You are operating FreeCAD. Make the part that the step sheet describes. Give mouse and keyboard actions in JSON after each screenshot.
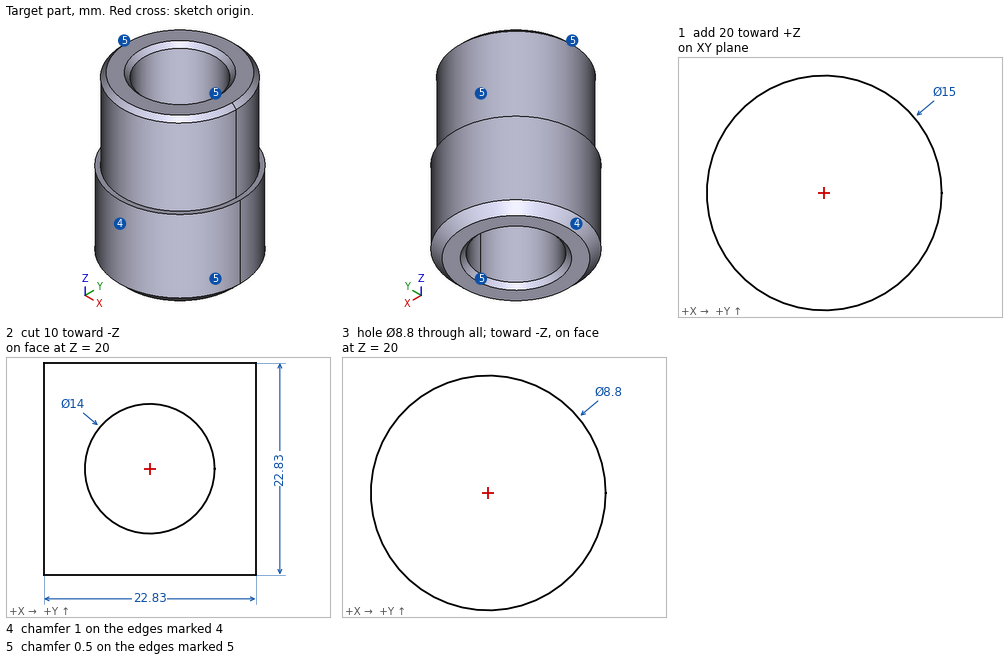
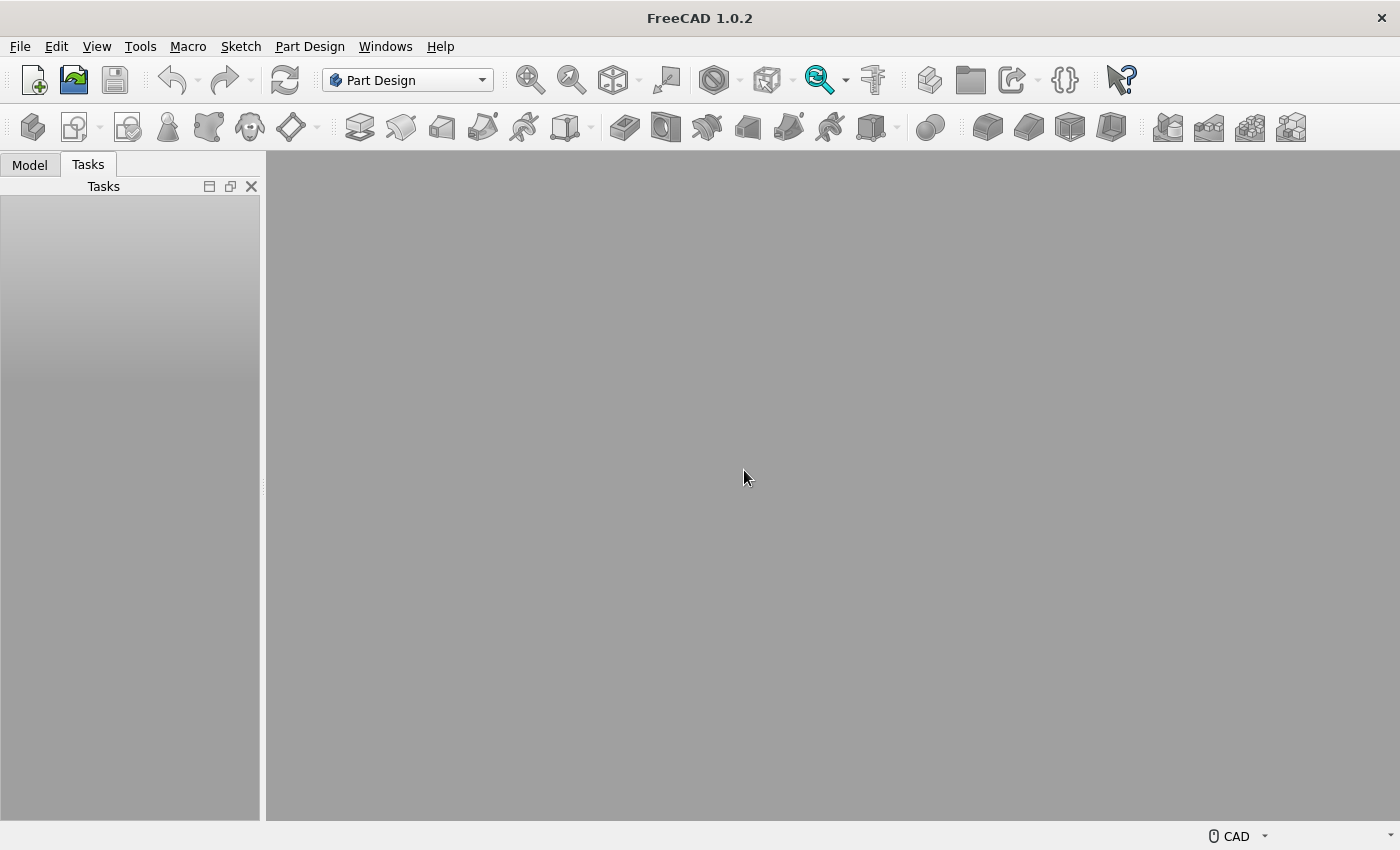
{"action": "left_click", "coordinate": [33, 80]}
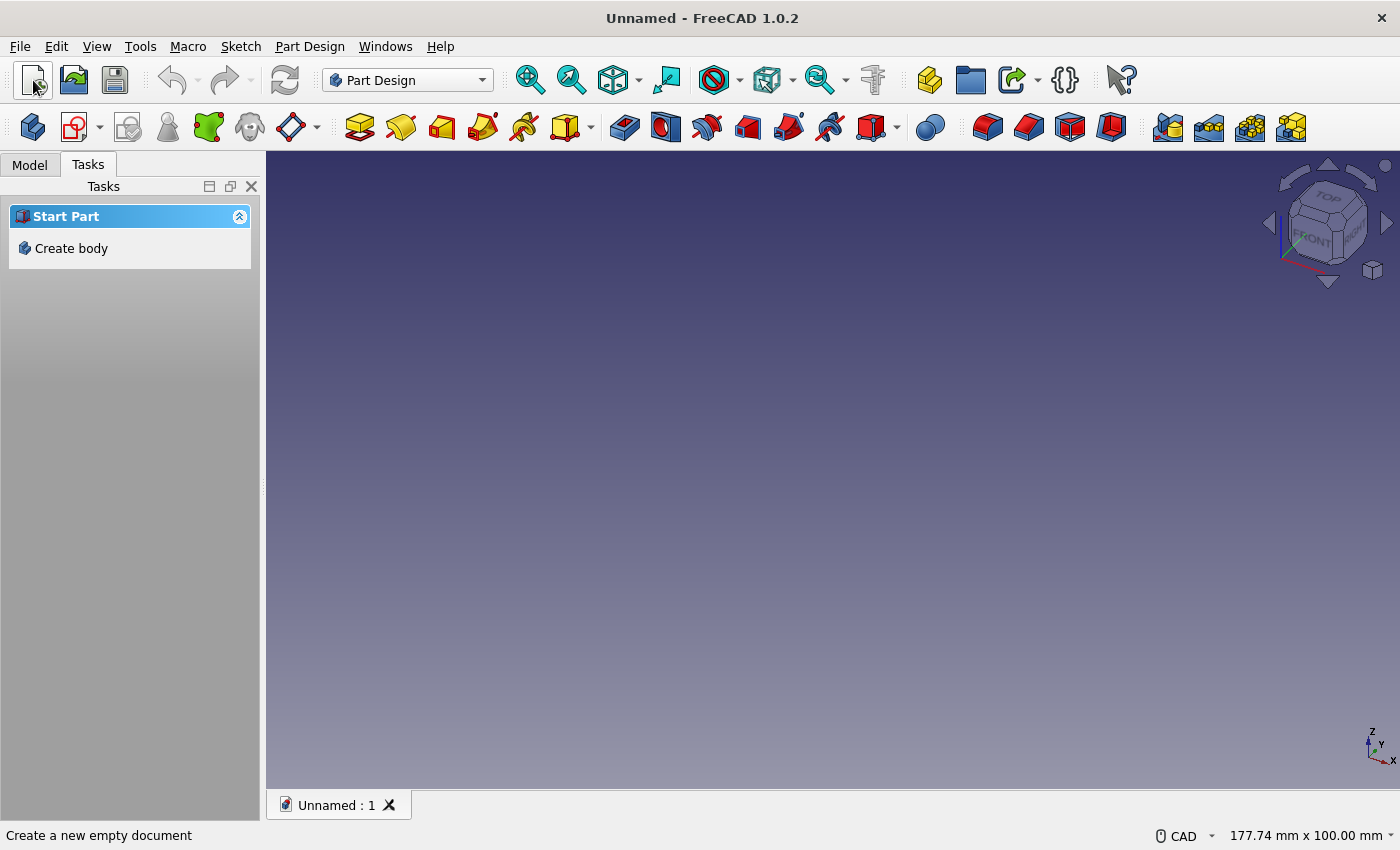
{"action": "left_click", "coordinate": [74, 128]}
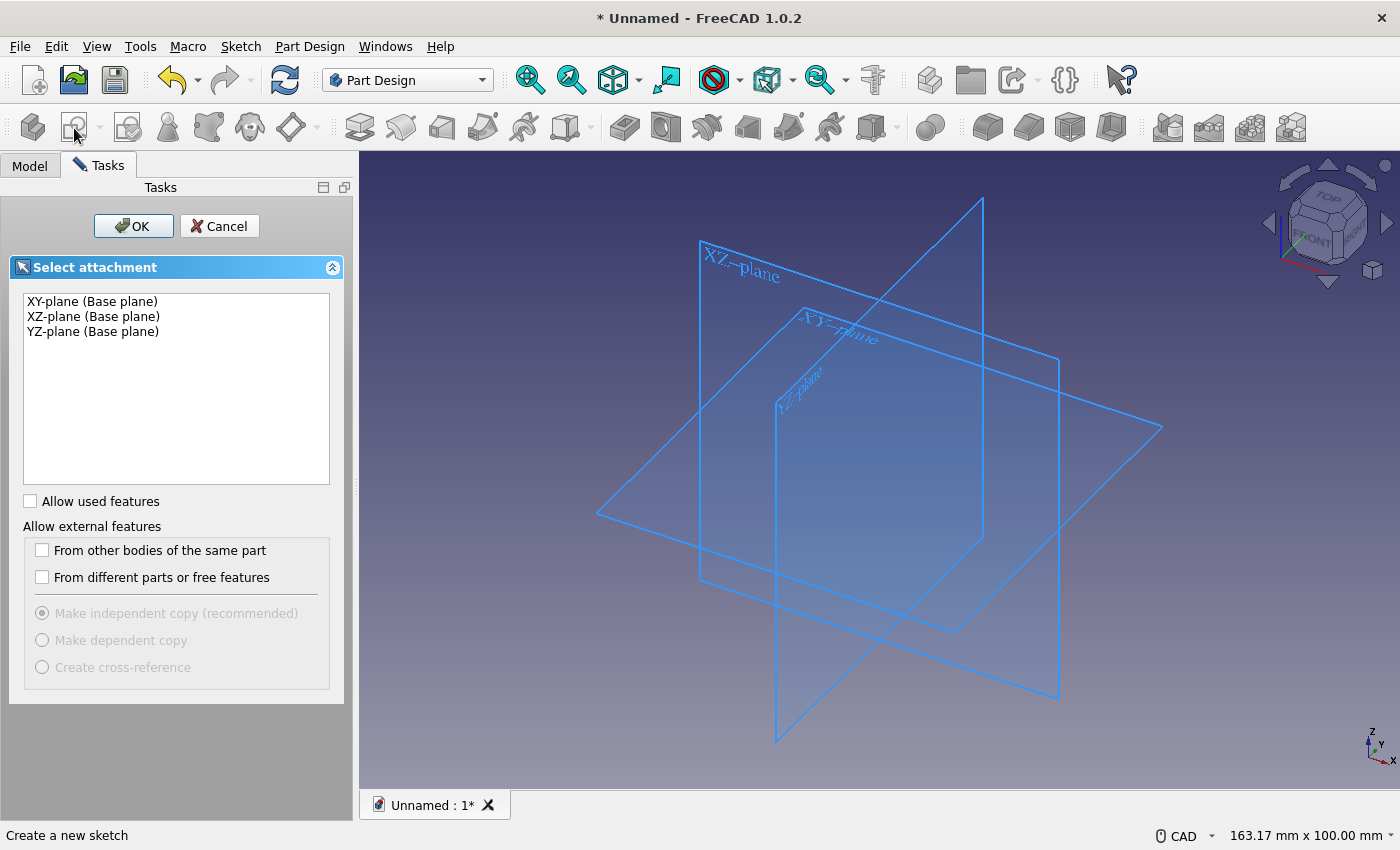
{"action": "left_click", "coordinate": [84, 302]}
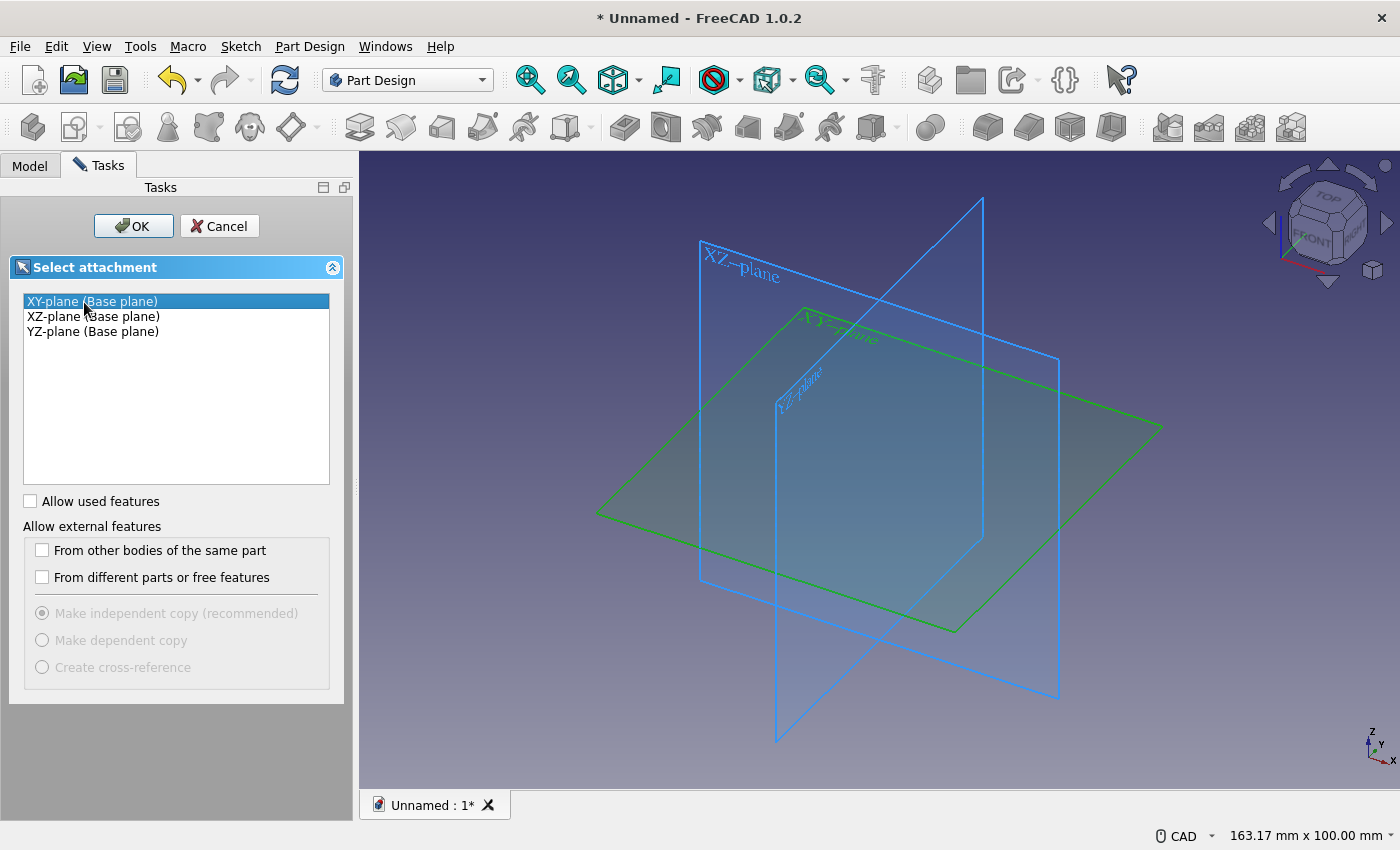
{"action": "left_click", "coordinate": [134, 226]}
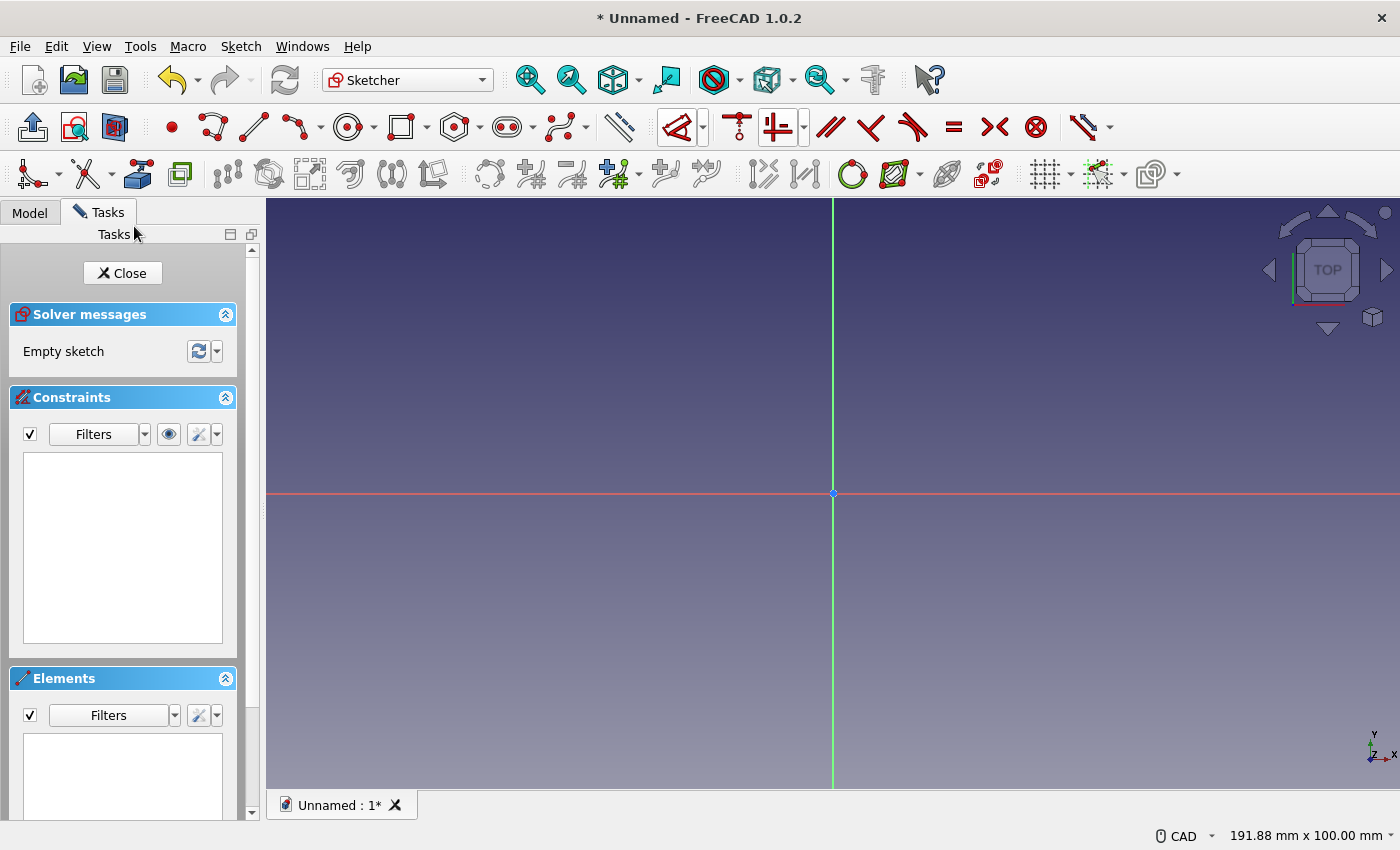
{"action": "scroll", "coordinate": [855, 494], "scroll_direction": "up", "scroll_amount": 7}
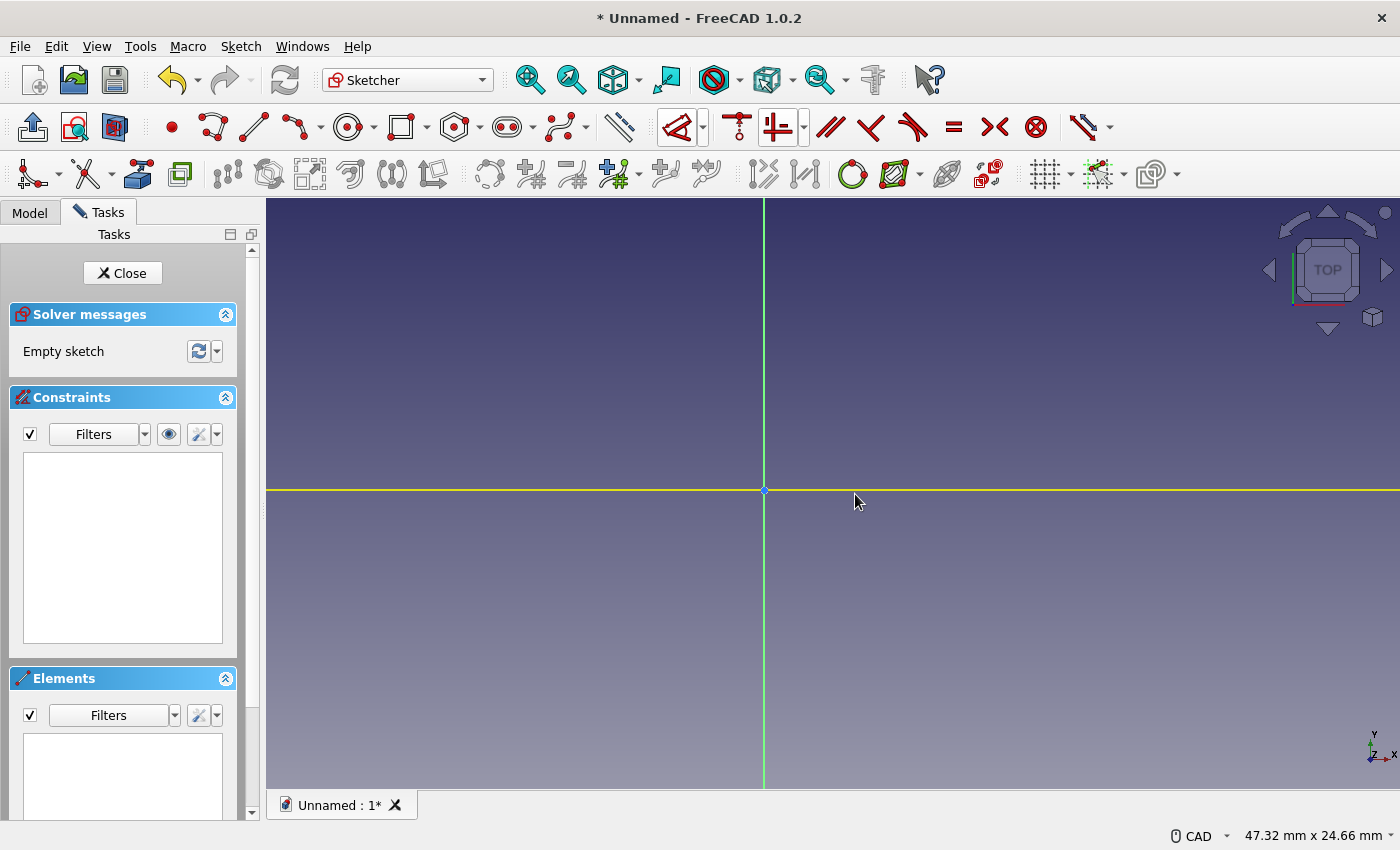
{"action": "key", "text": "g c"}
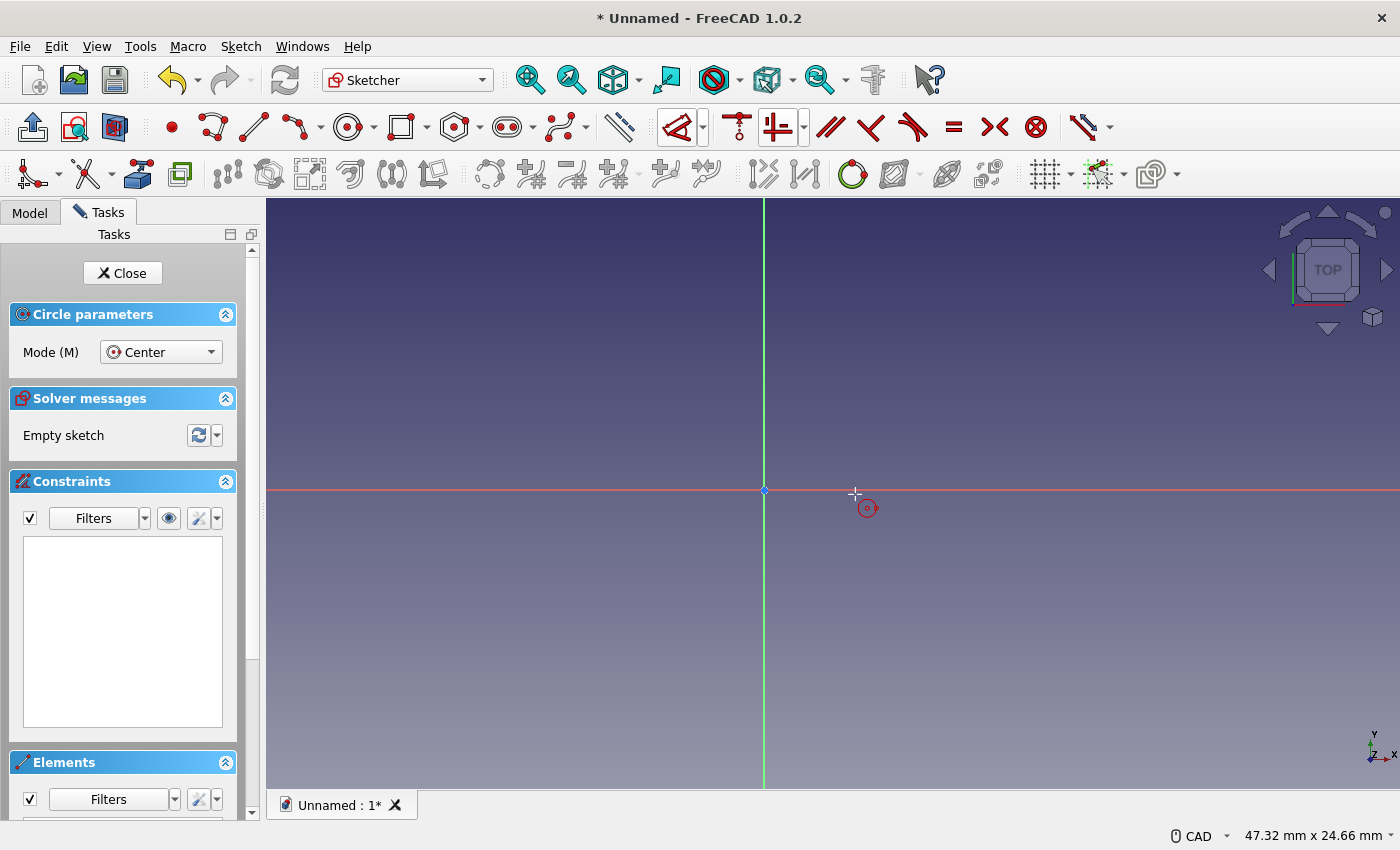
{"action": "left_click", "coordinate": [764, 490]}
{"action": "mouse_move", "coordinate": [891, 363]}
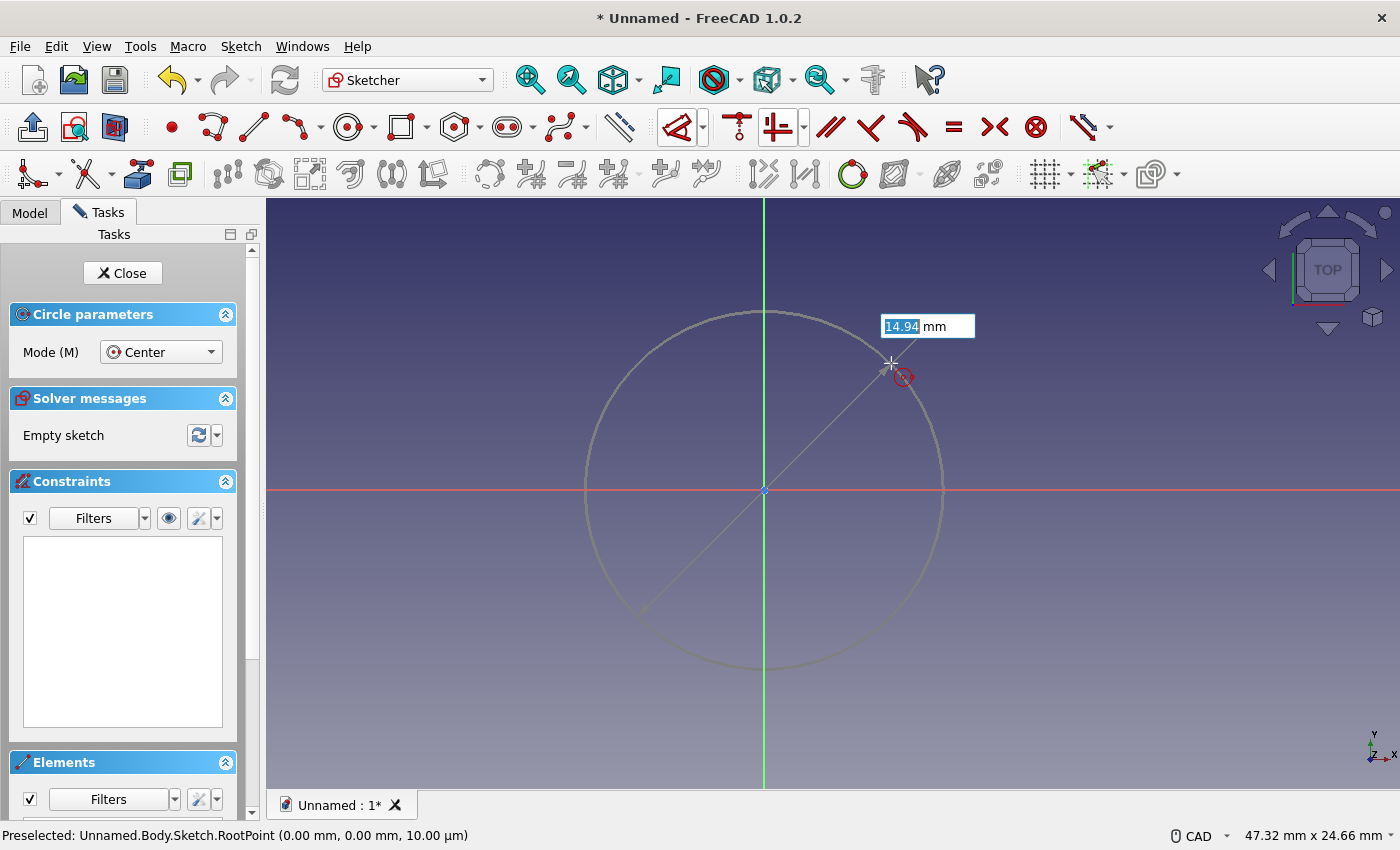
{"action": "type", "text": "15"}
{"action": "key", "text": "Return"}
{"action": "key", "text": "Escape"}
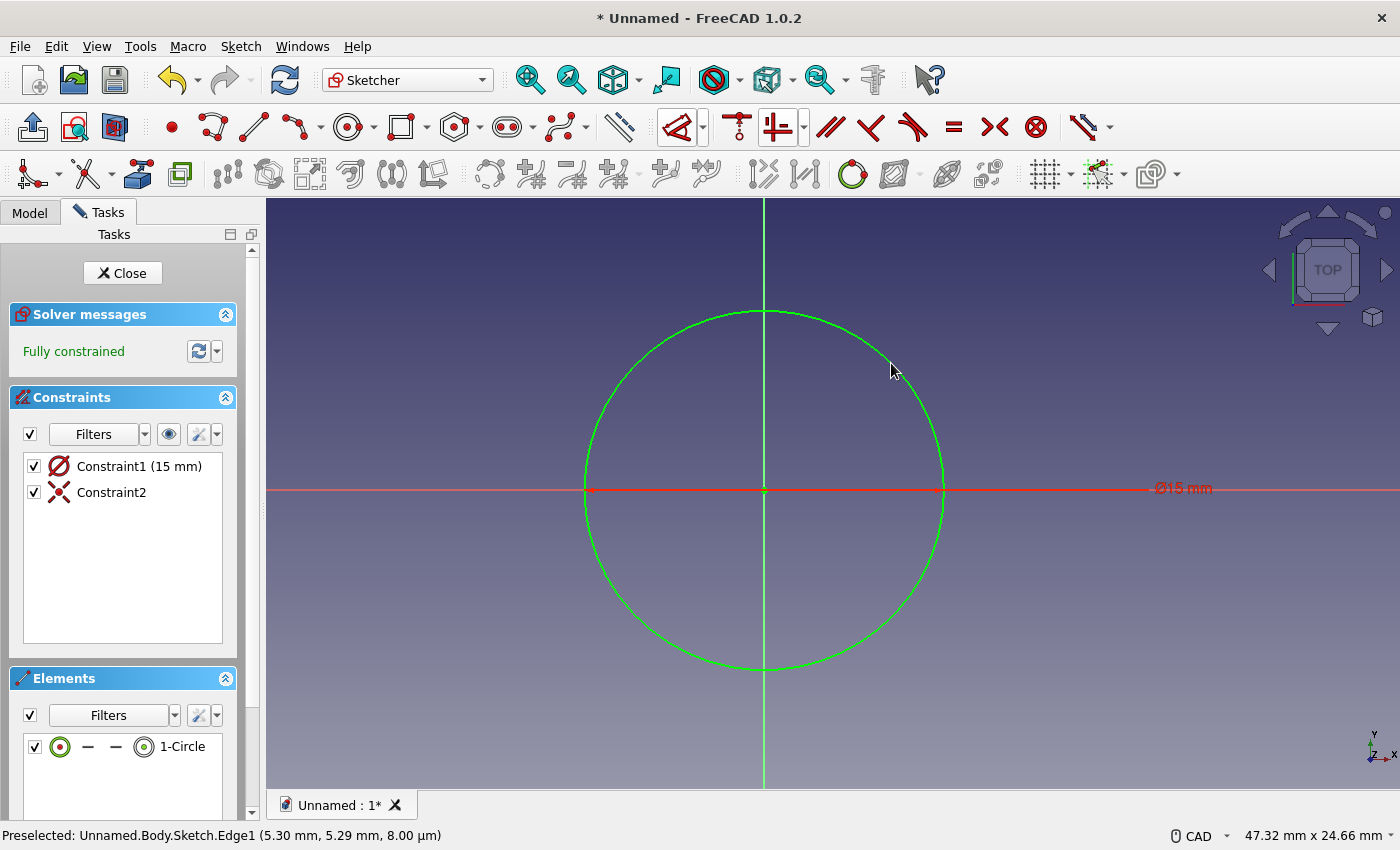
{"action": "left_click", "coordinate": [123, 273]}